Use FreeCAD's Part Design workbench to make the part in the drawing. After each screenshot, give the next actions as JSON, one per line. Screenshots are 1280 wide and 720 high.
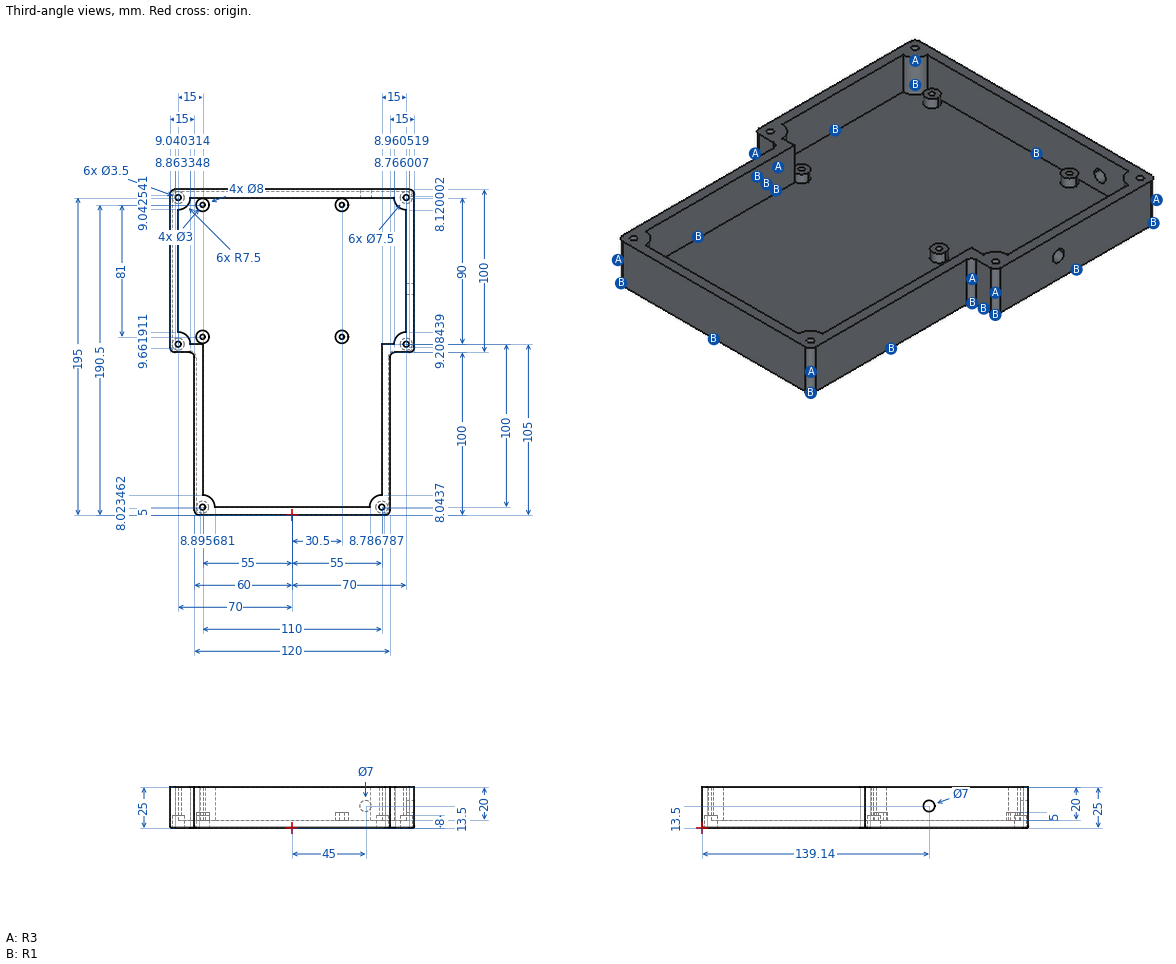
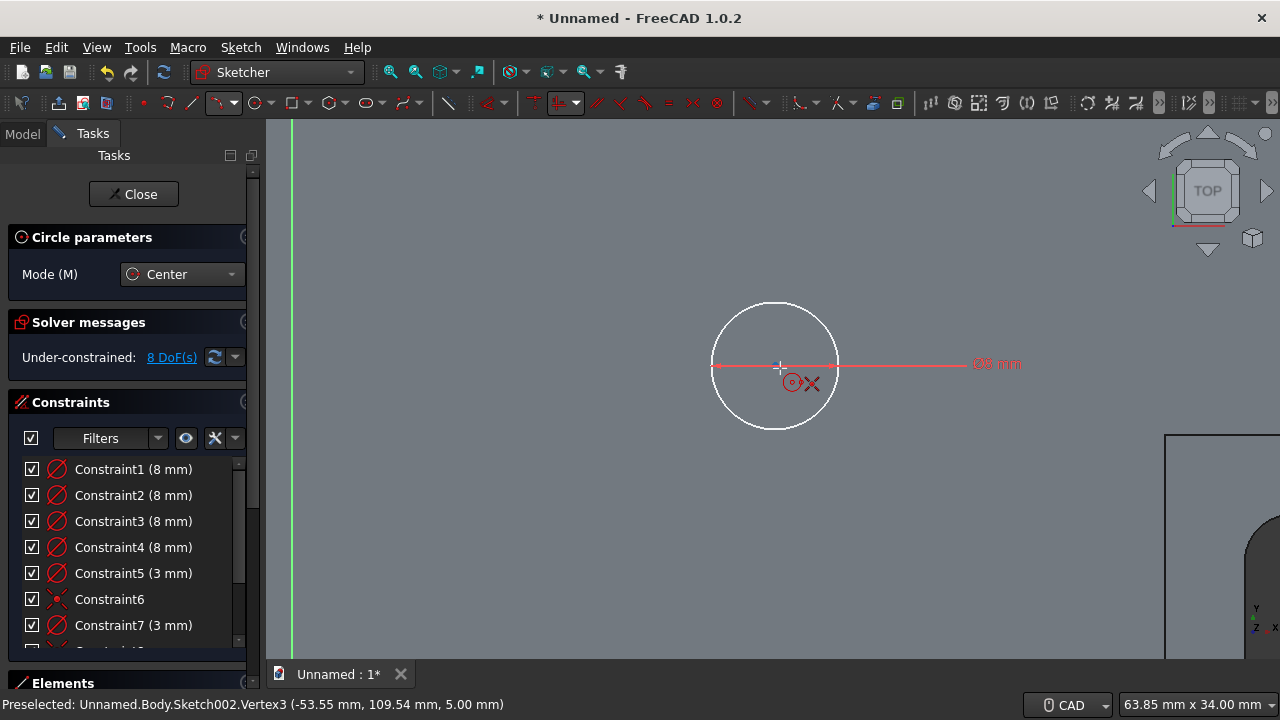
{"action": "scroll", "coordinate": [780, 368], "scroll_direction": "down", "scroll_amount": 11}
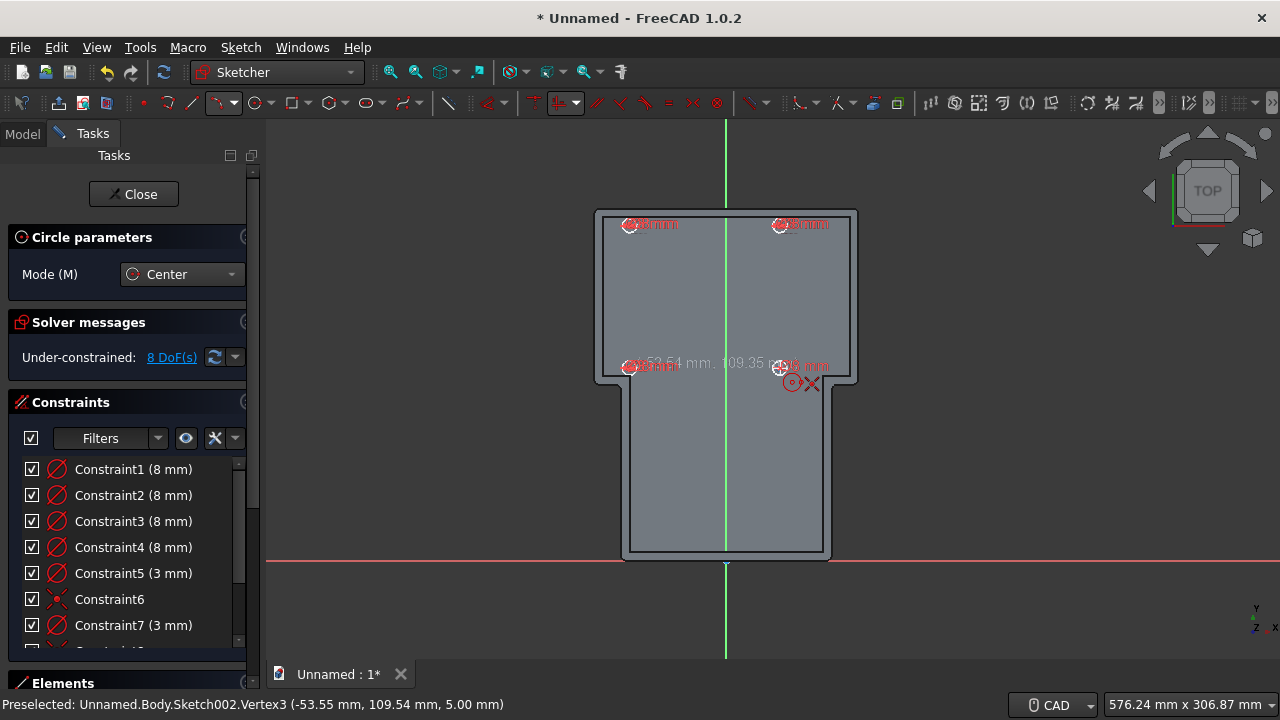
{"action": "scroll", "coordinate": [780, 368], "scroll_direction": "up", "scroll_amount": 5}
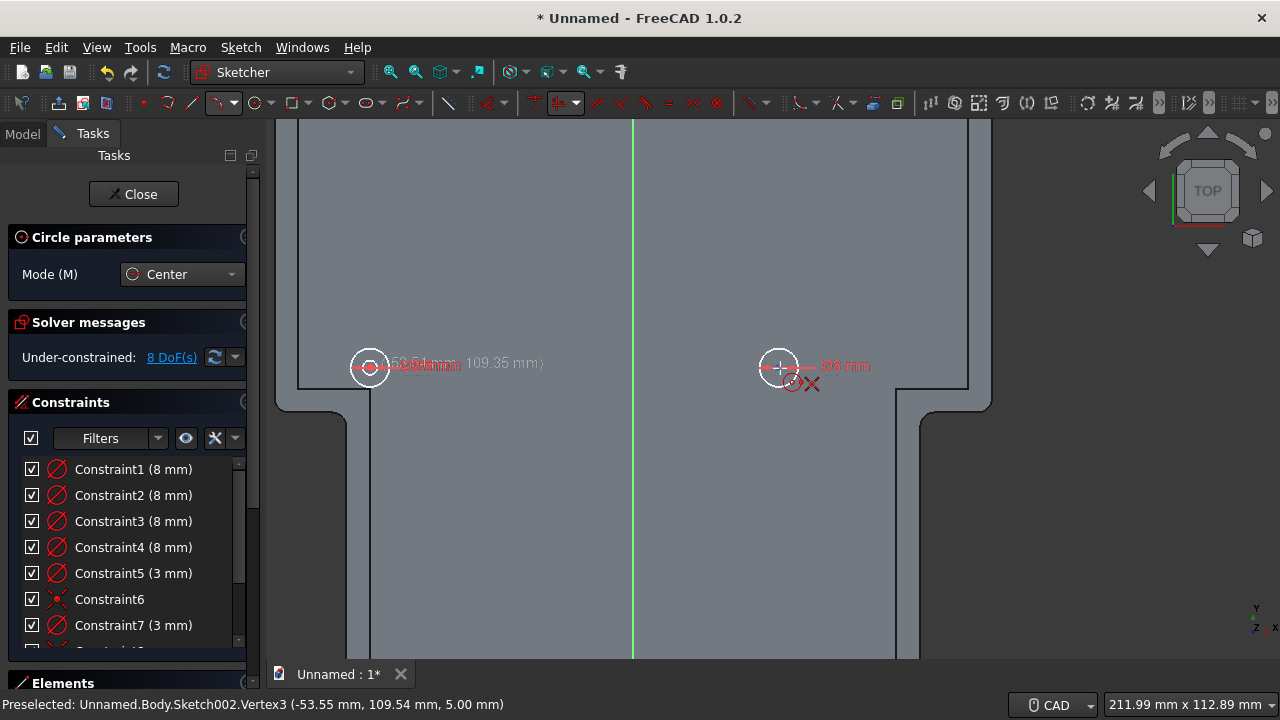
{"action": "left_click", "coordinate": [779, 368]}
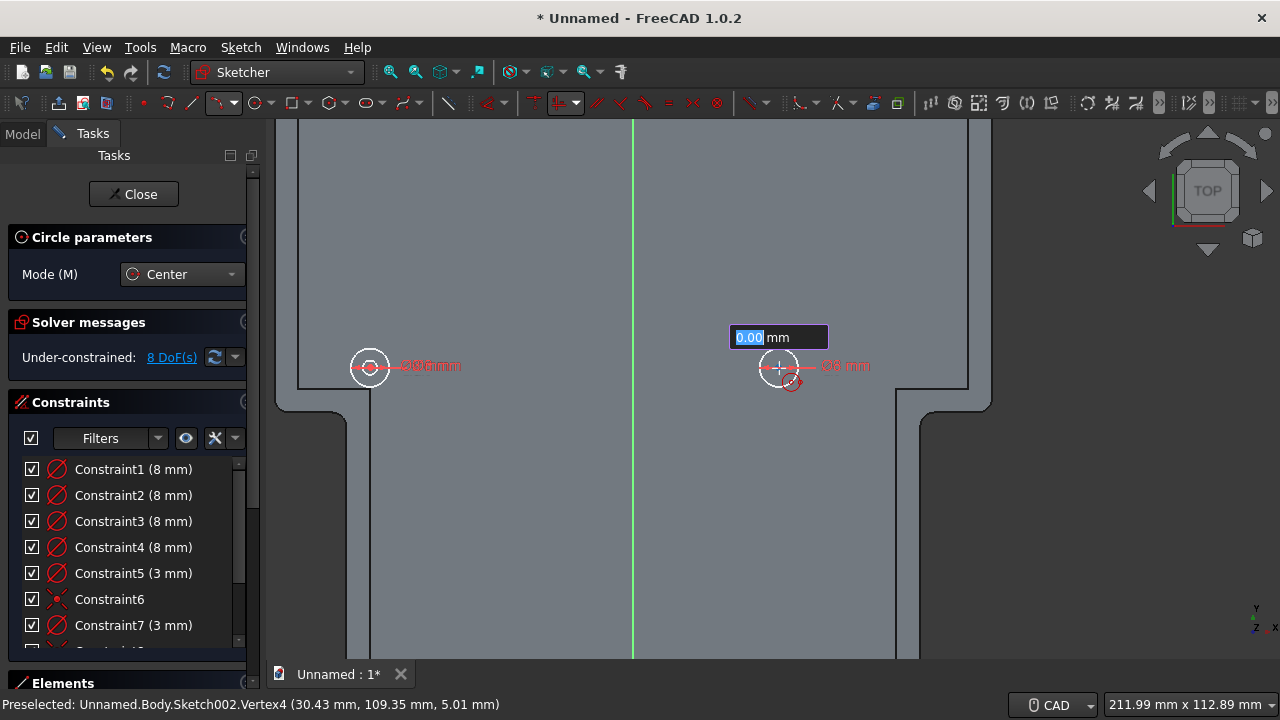
{"action": "scroll", "coordinate": [786, 365], "scroll_direction": "up", "scroll_amount": 4}
{"action": "mouse_move", "coordinate": [785, 363]}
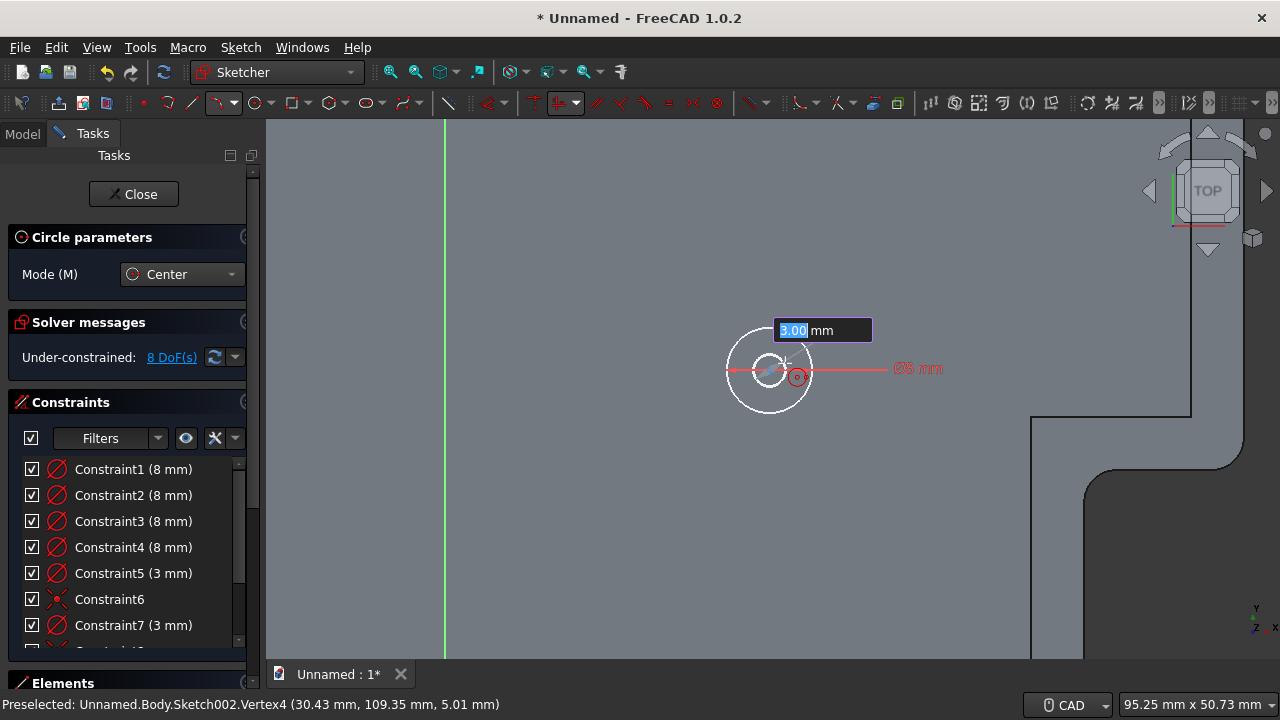
{"action": "type", "text": "3"}
{"action": "key", "text": "Return"}
{"action": "key", "text": "Escape"}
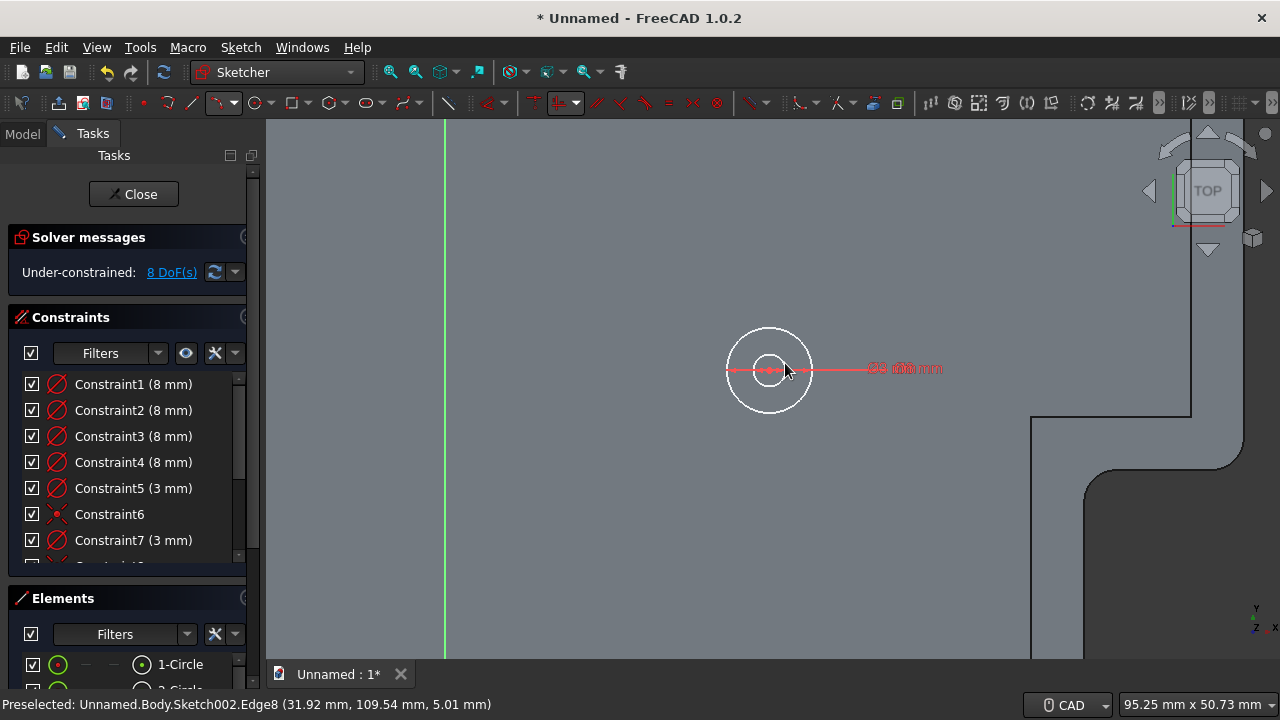
{"action": "scroll", "coordinate": [782, 367], "scroll_direction": "down", "scroll_amount": 9}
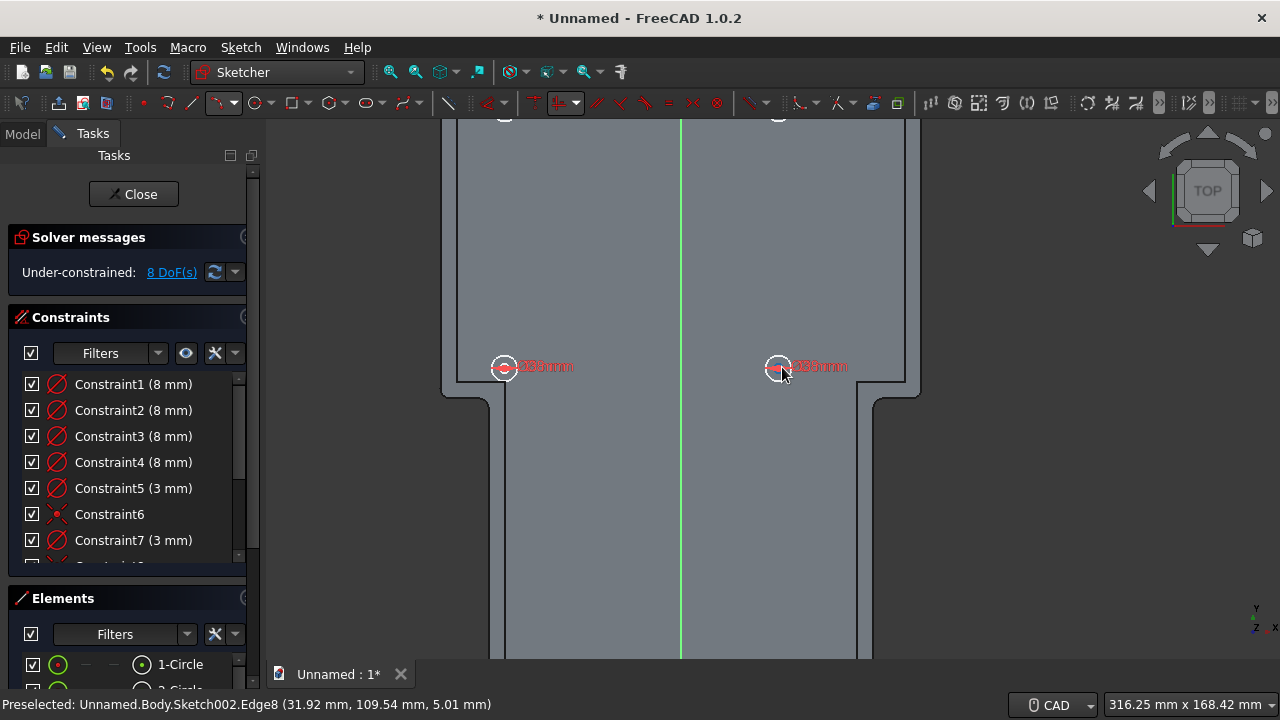
{"action": "left_click", "coordinate": [630, 225]}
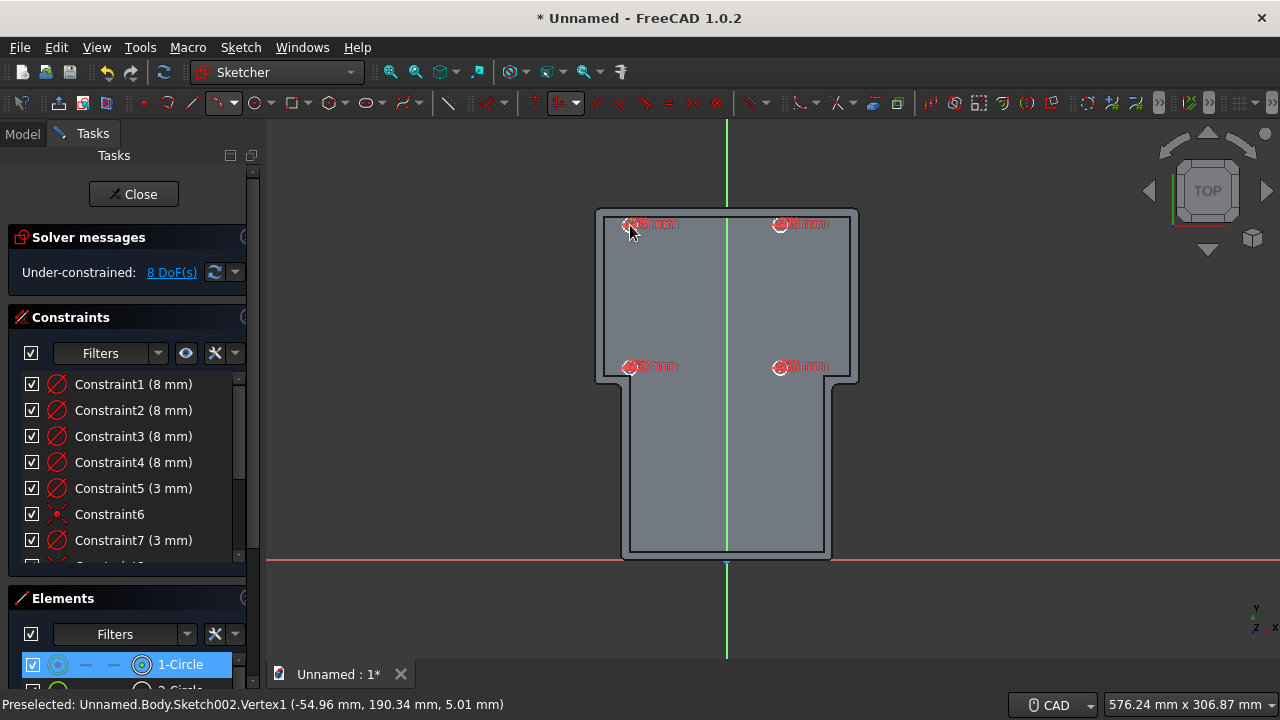
{"action": "left_click", "coordinate": [780, 225]}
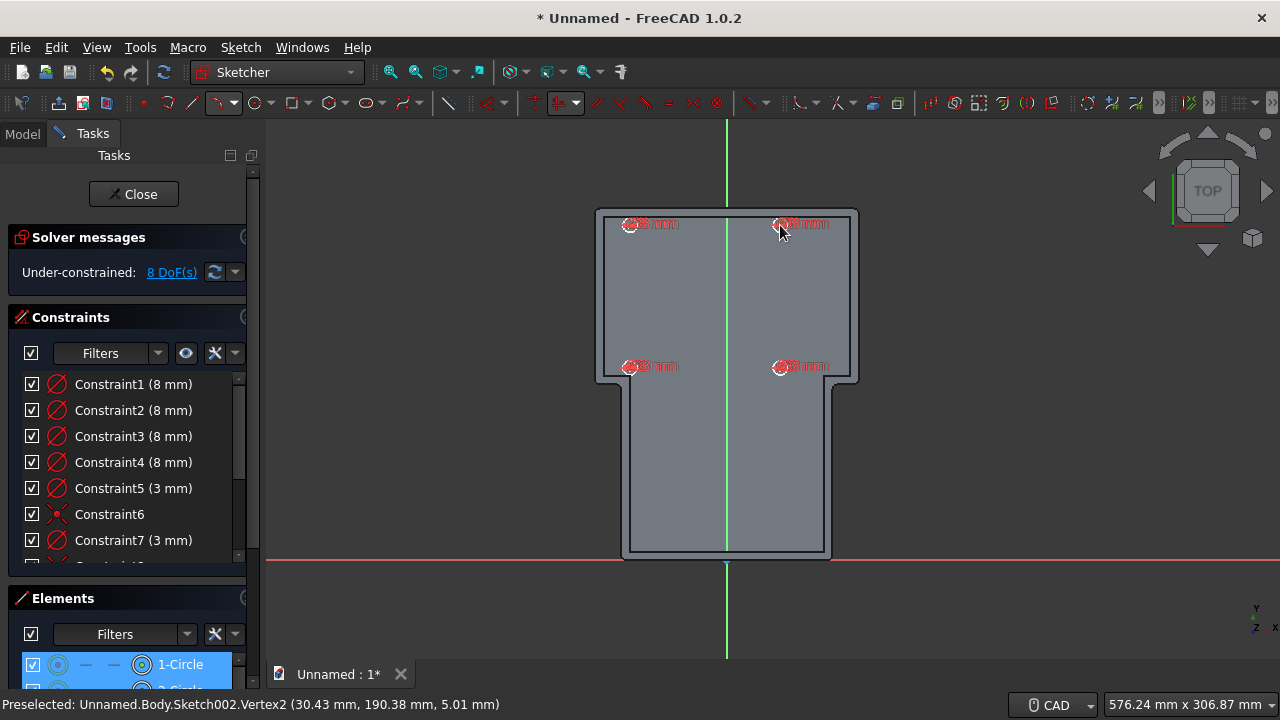
{"action": "key", "text": "h"}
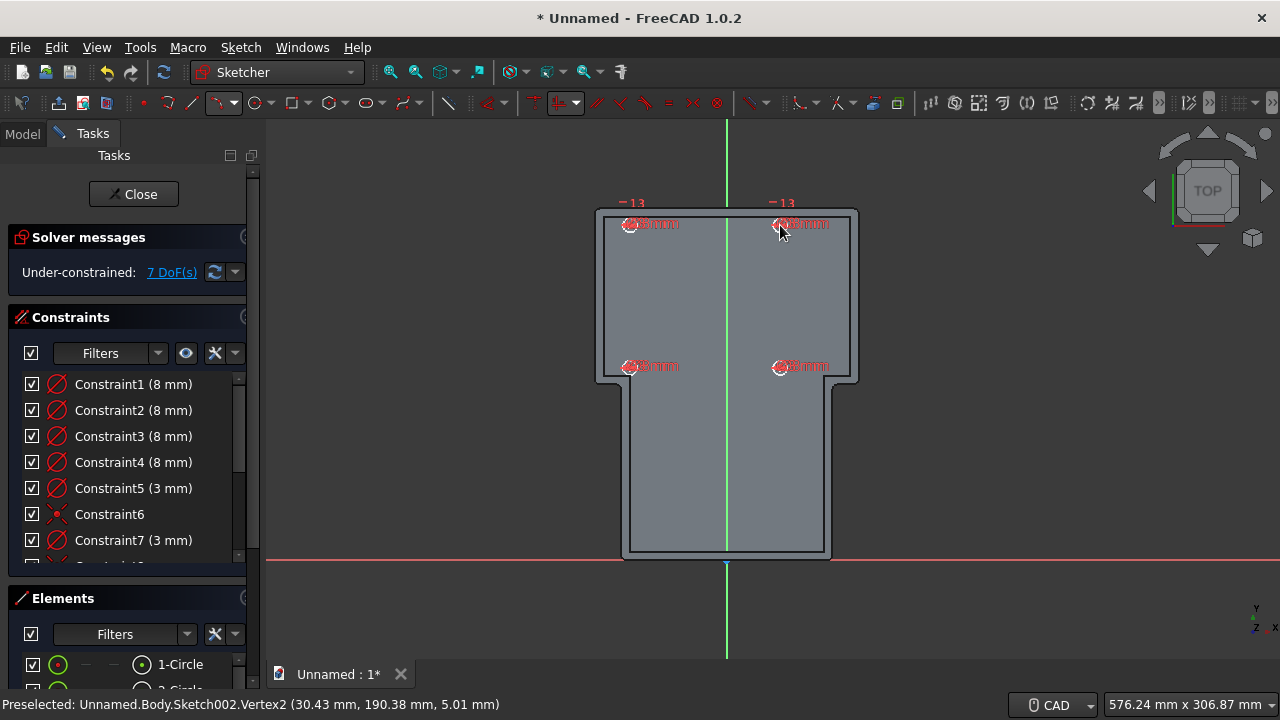
{"action": "left_click", "coordinate": [630, 225]}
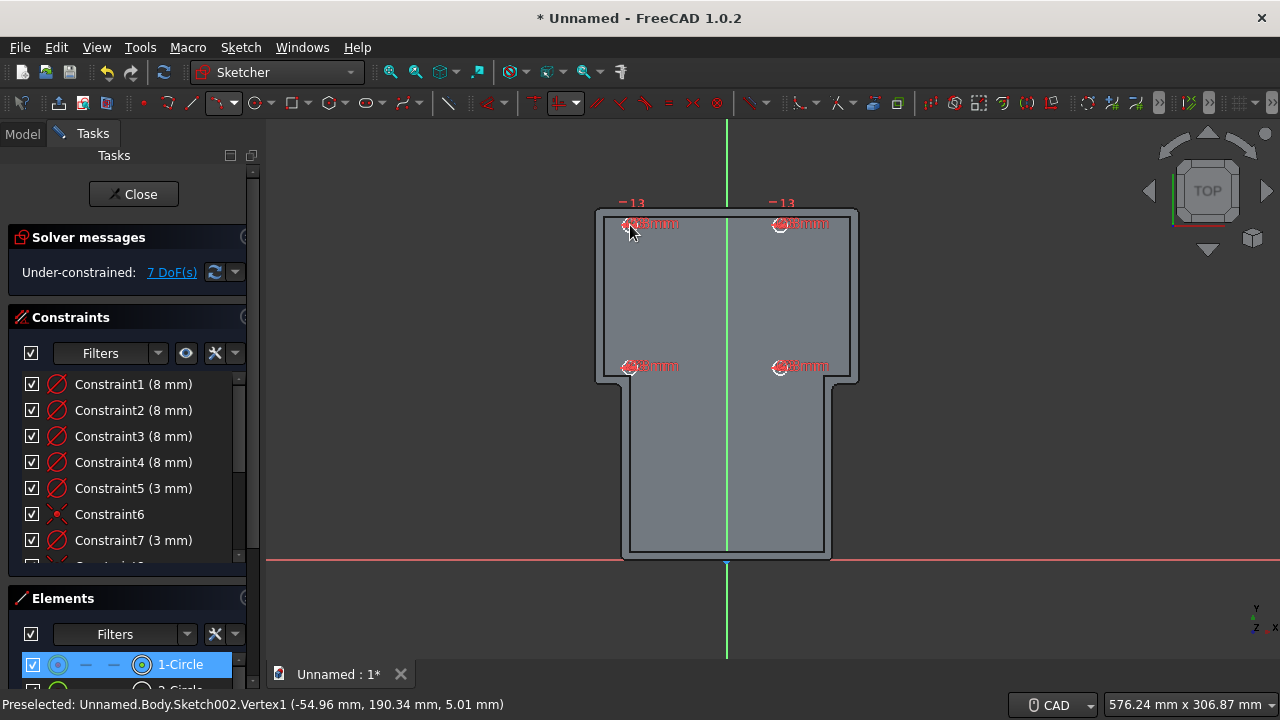
{"action": "left_click", "coordinate": [630, 368]}